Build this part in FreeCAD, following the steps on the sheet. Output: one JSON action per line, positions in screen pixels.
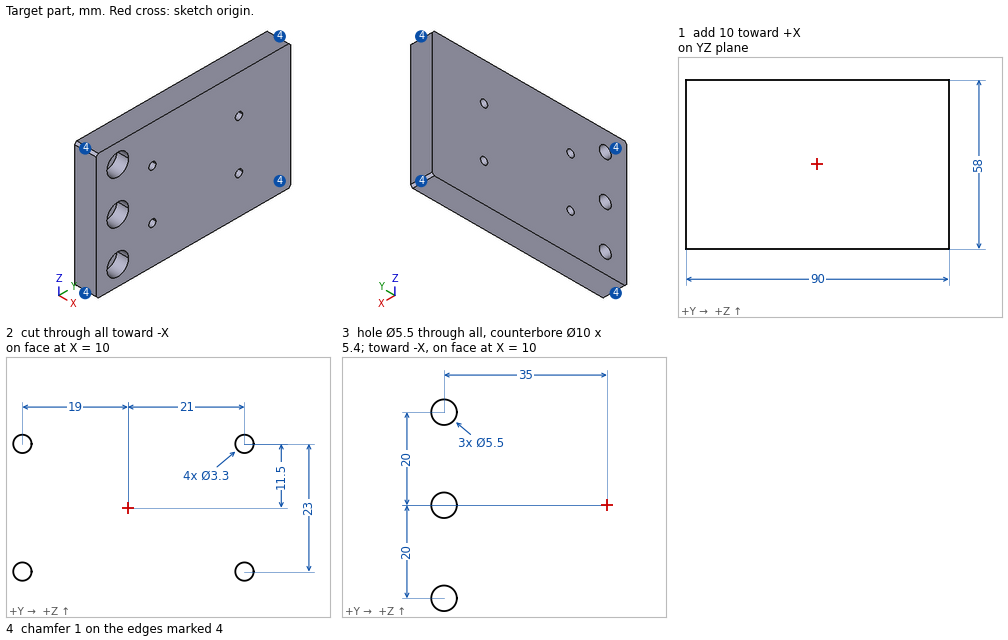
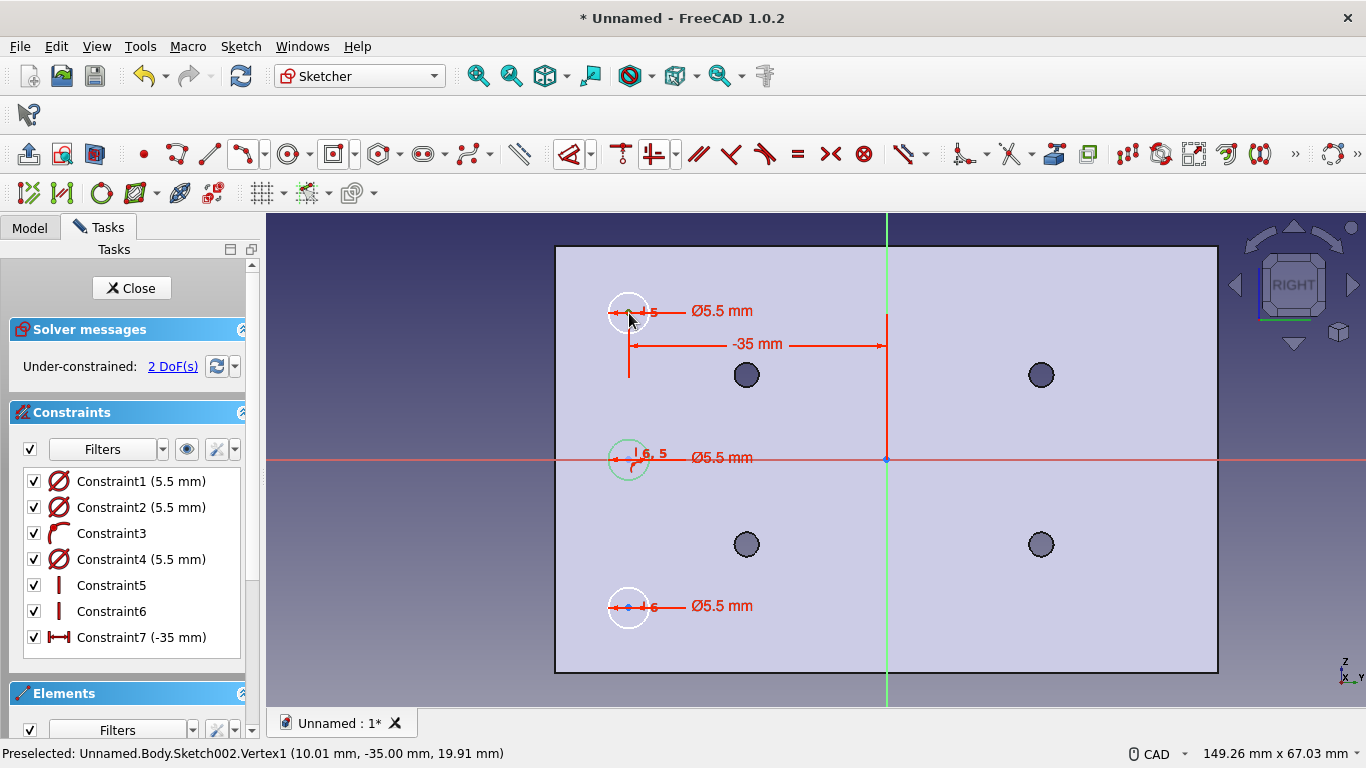
{"action": "key", "text": "i"}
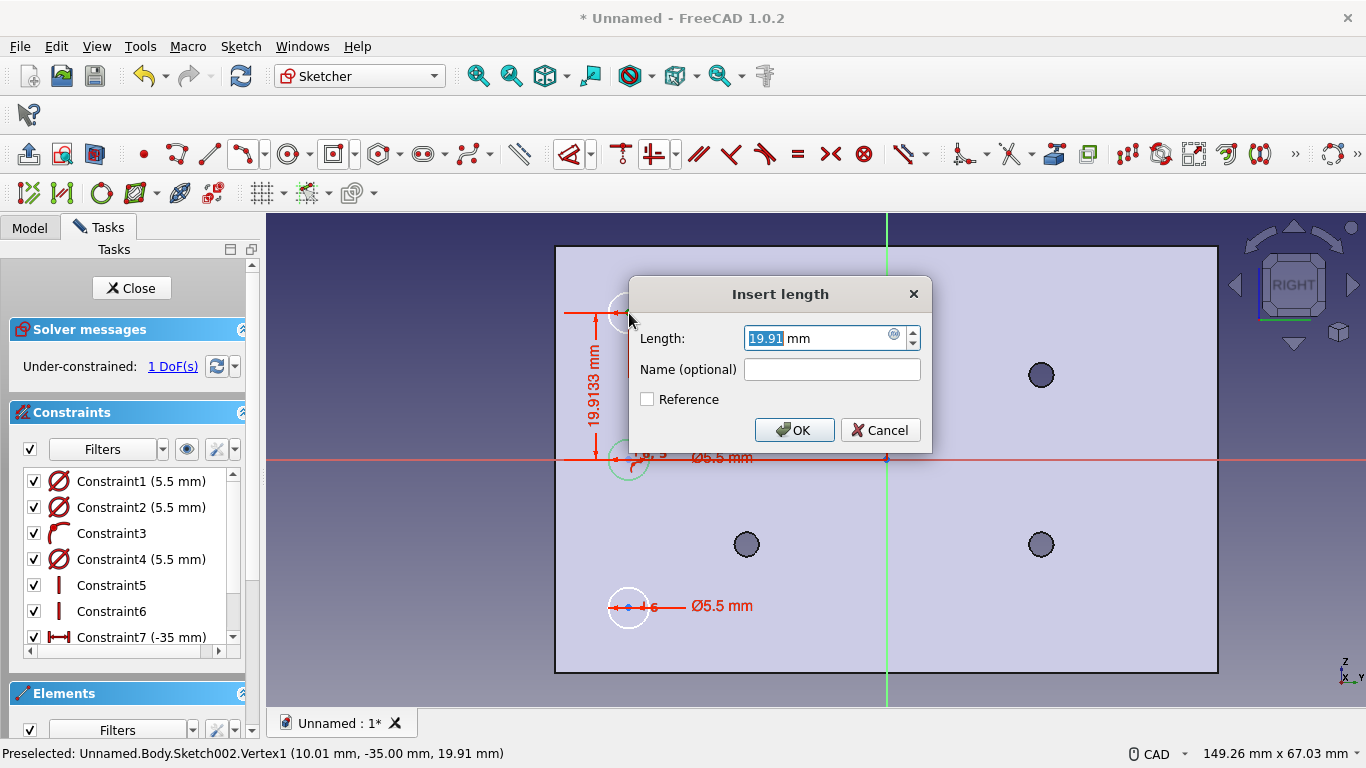
{"action": "type", "text": "20"}
{"action": "key", "text": "Return"}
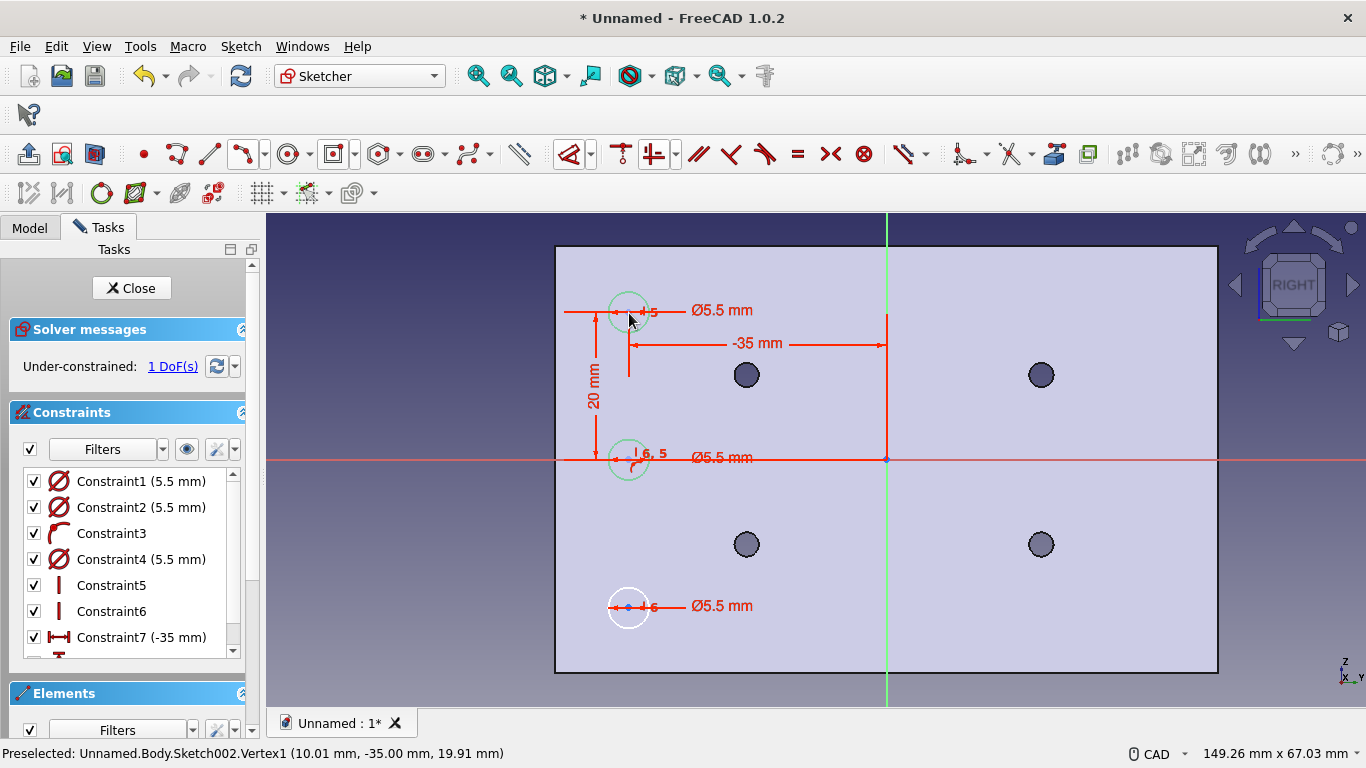
{"action": "left_click", "coordinate": [629, 608]}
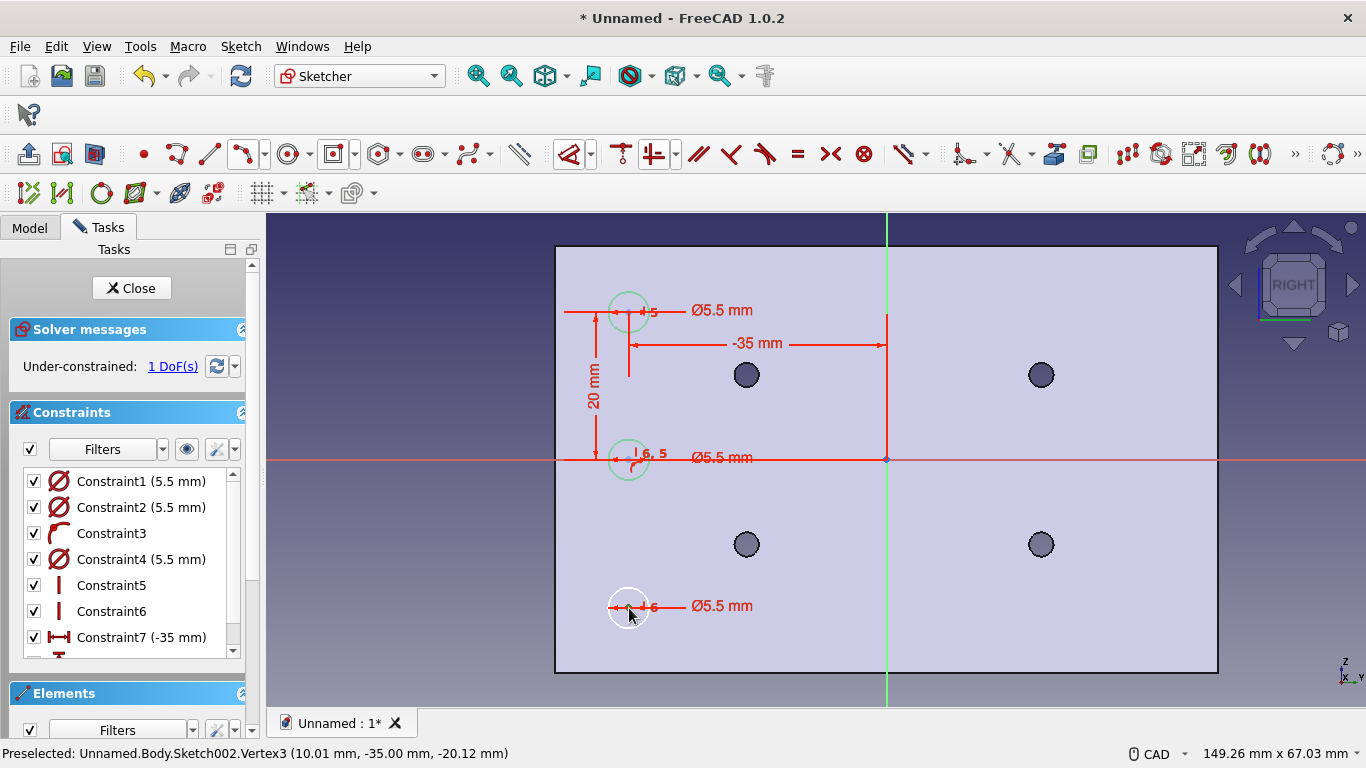
{"action": "left_click", "coordinate": [590, 154]}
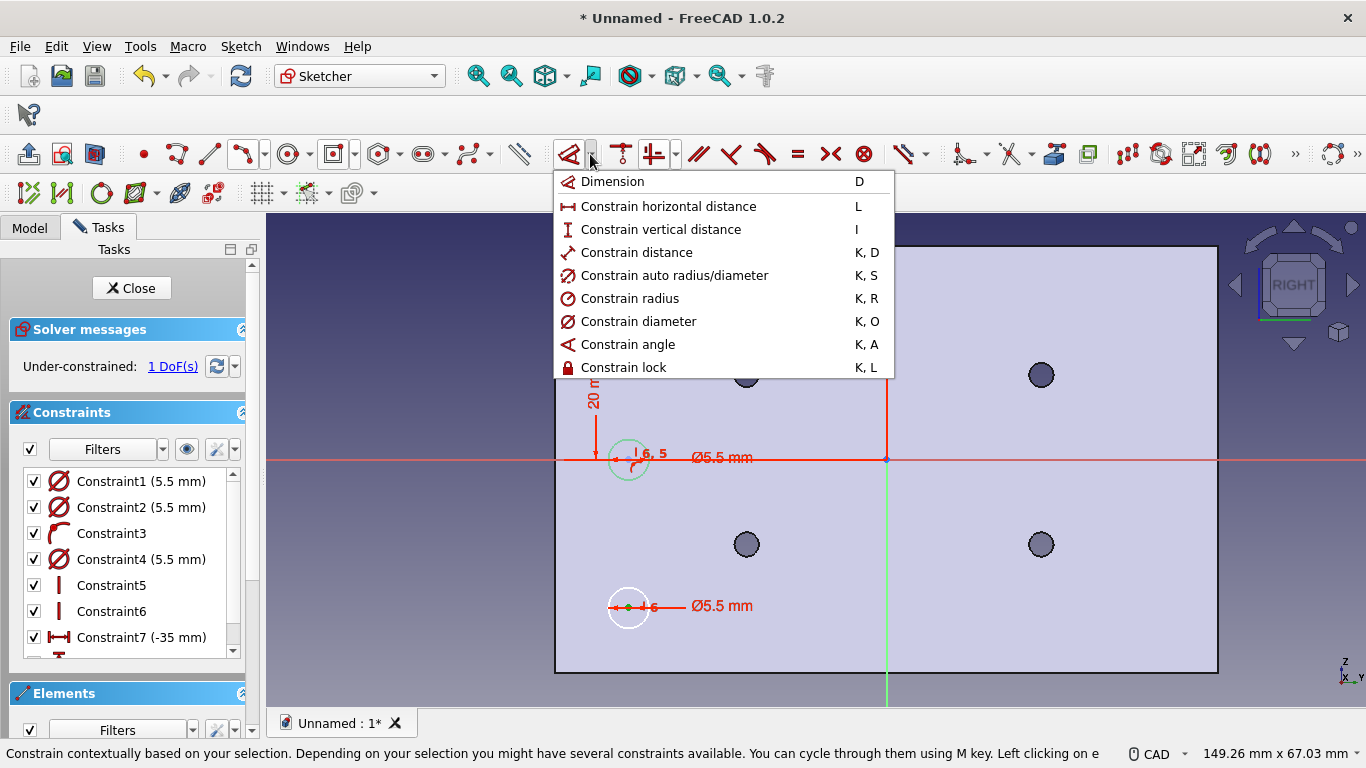
{"action": "left_click", "coordinate": [724, 230]}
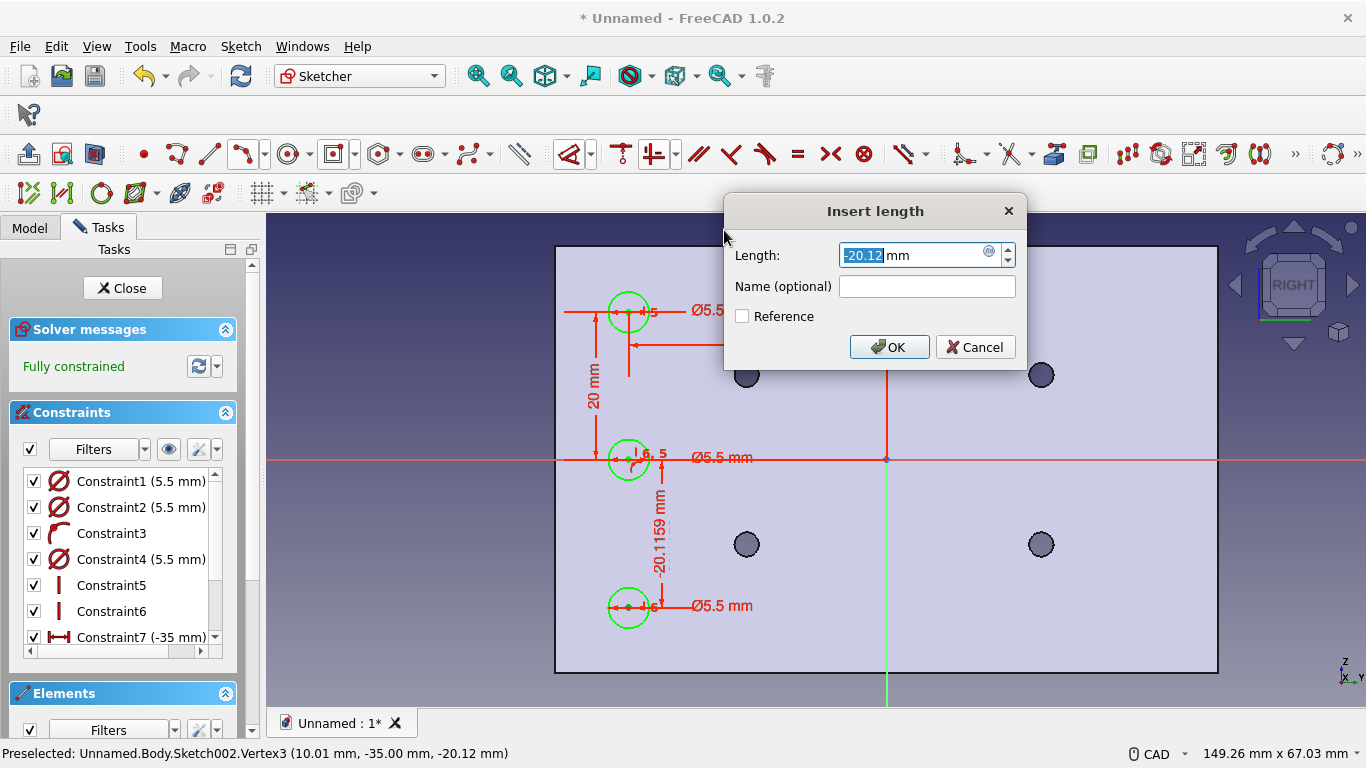
{"action": "type", "text": "-20"}
{"action": "key", "text": "Return"}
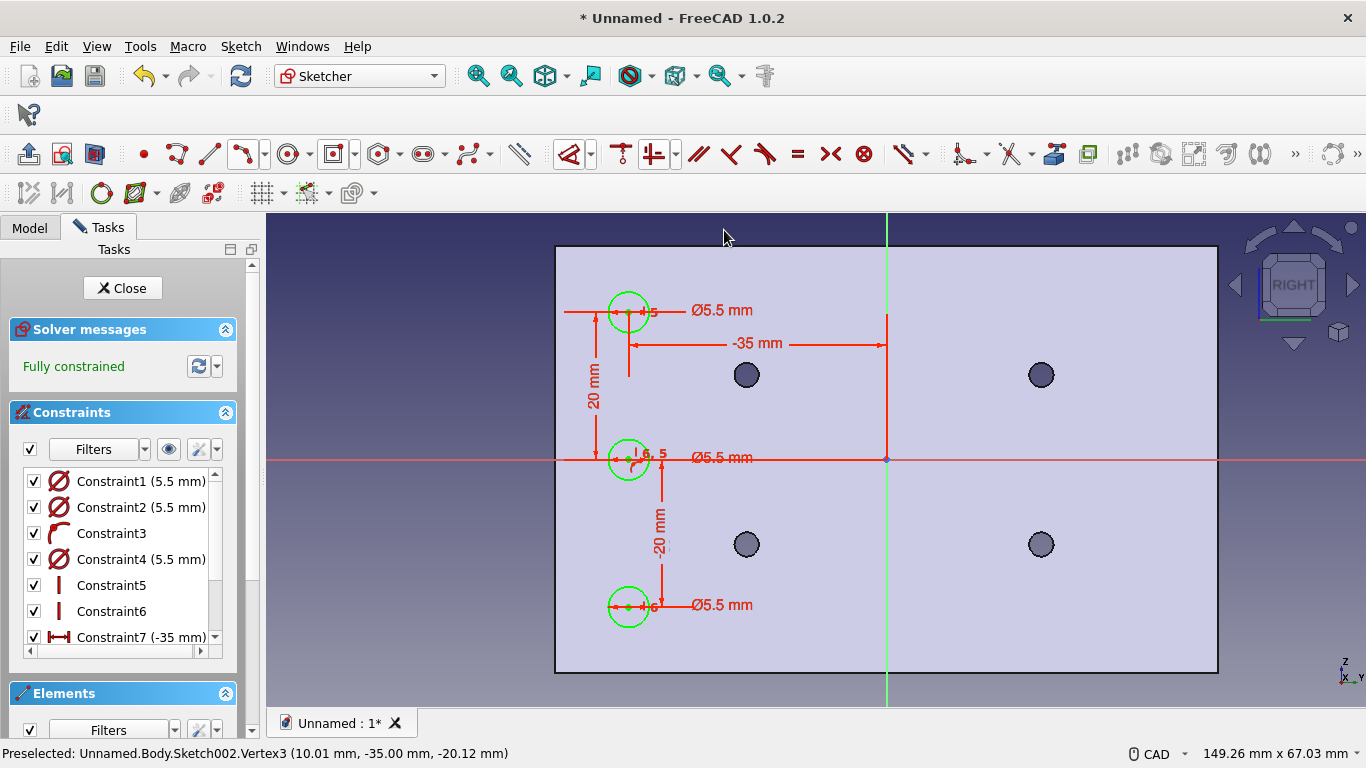
{"action": "left_click", "coordinate": [123, 288]}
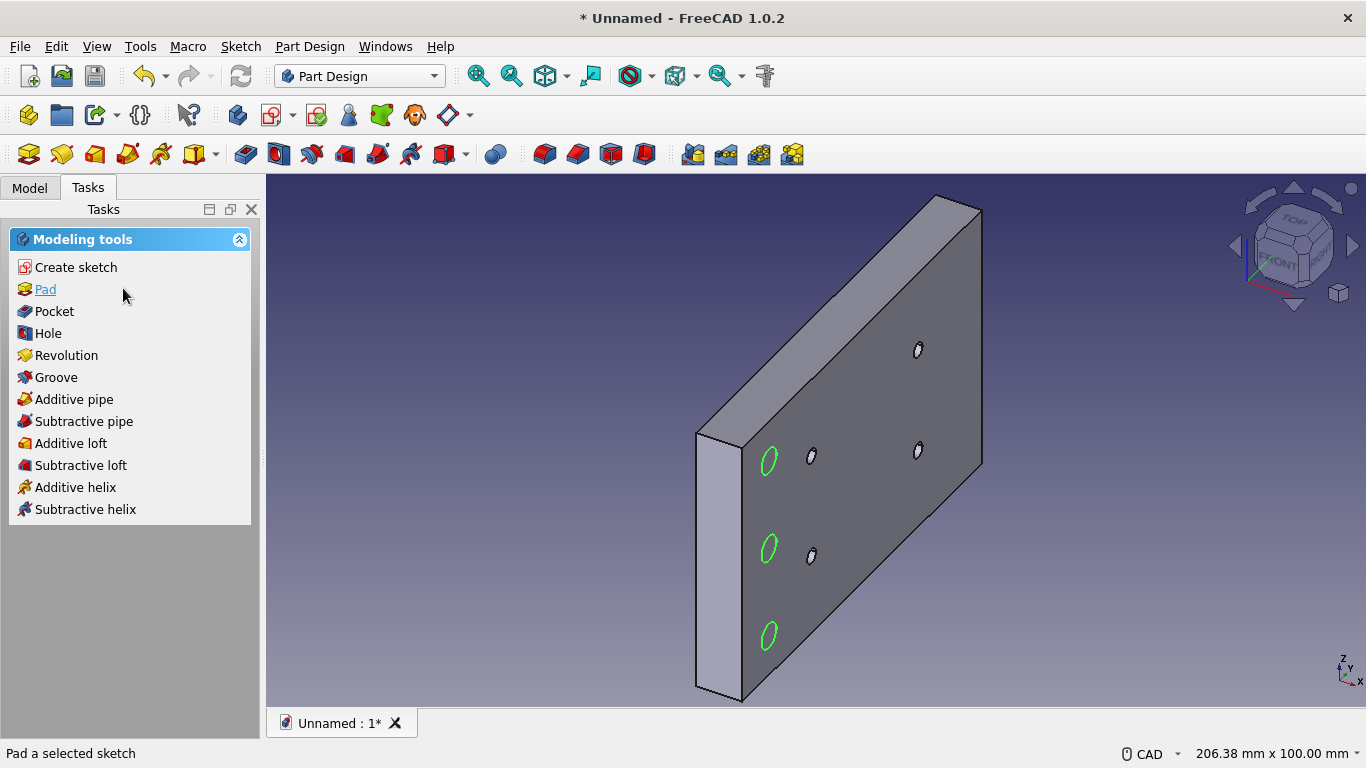
{"action": "left_click", "coordinate": [279, 154]}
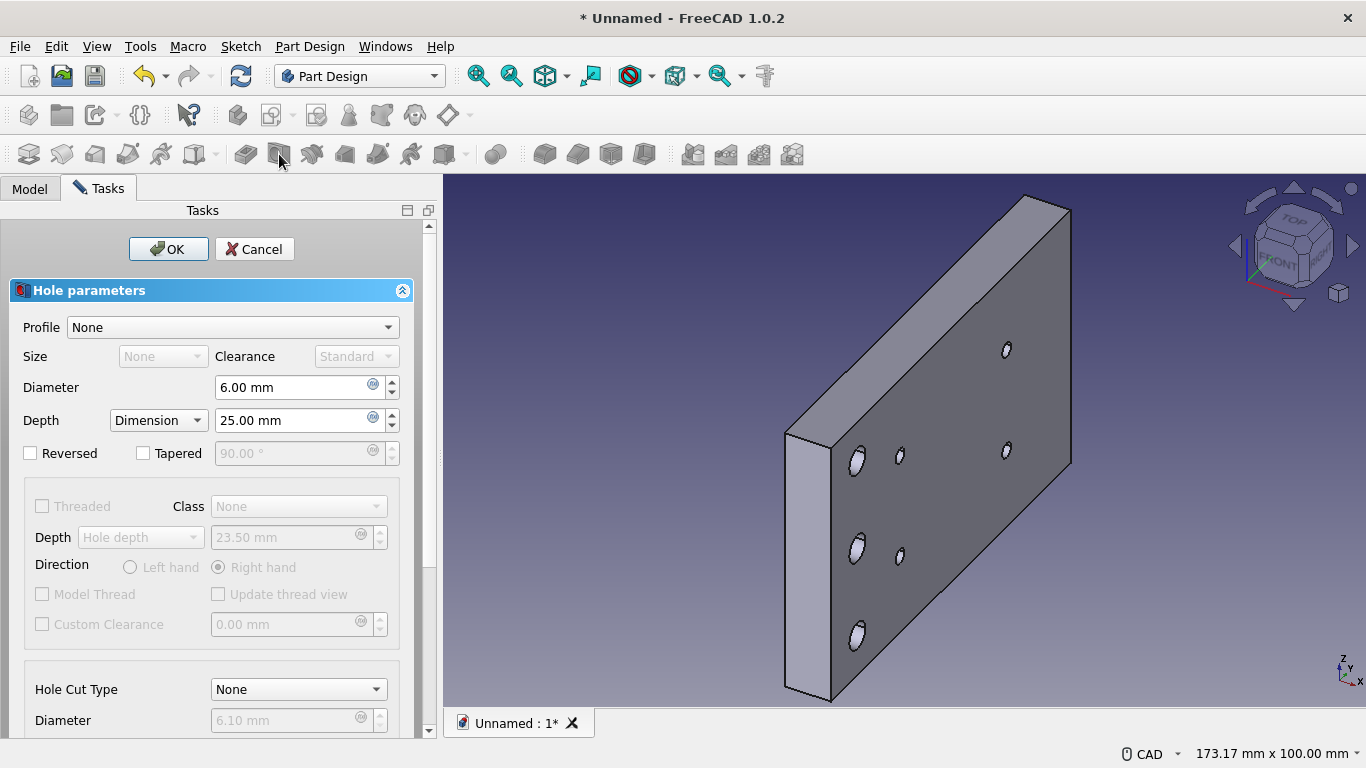
{"action": "triple_click", "coordinate": [300, 388]}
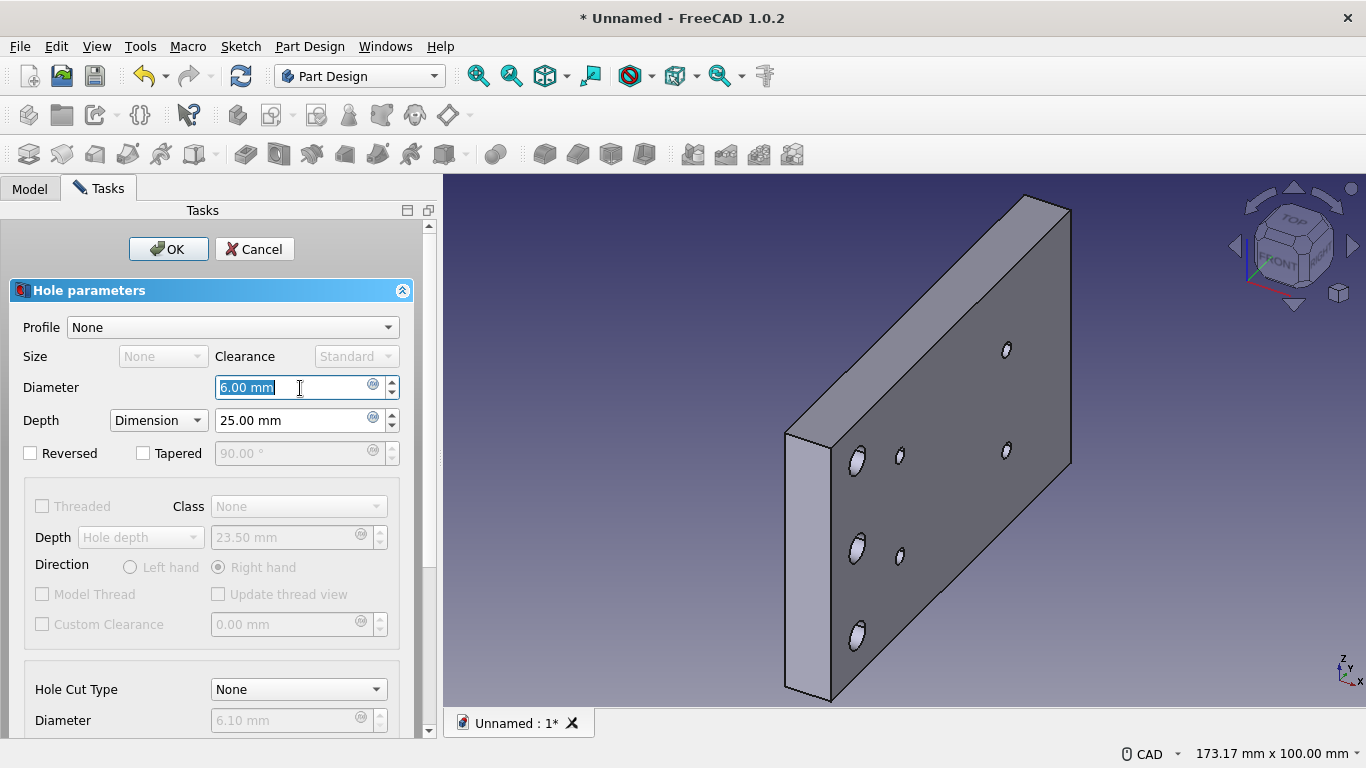
{"action": "type", "text": "5.5"}
{"action": "key", "text": "Tab"}